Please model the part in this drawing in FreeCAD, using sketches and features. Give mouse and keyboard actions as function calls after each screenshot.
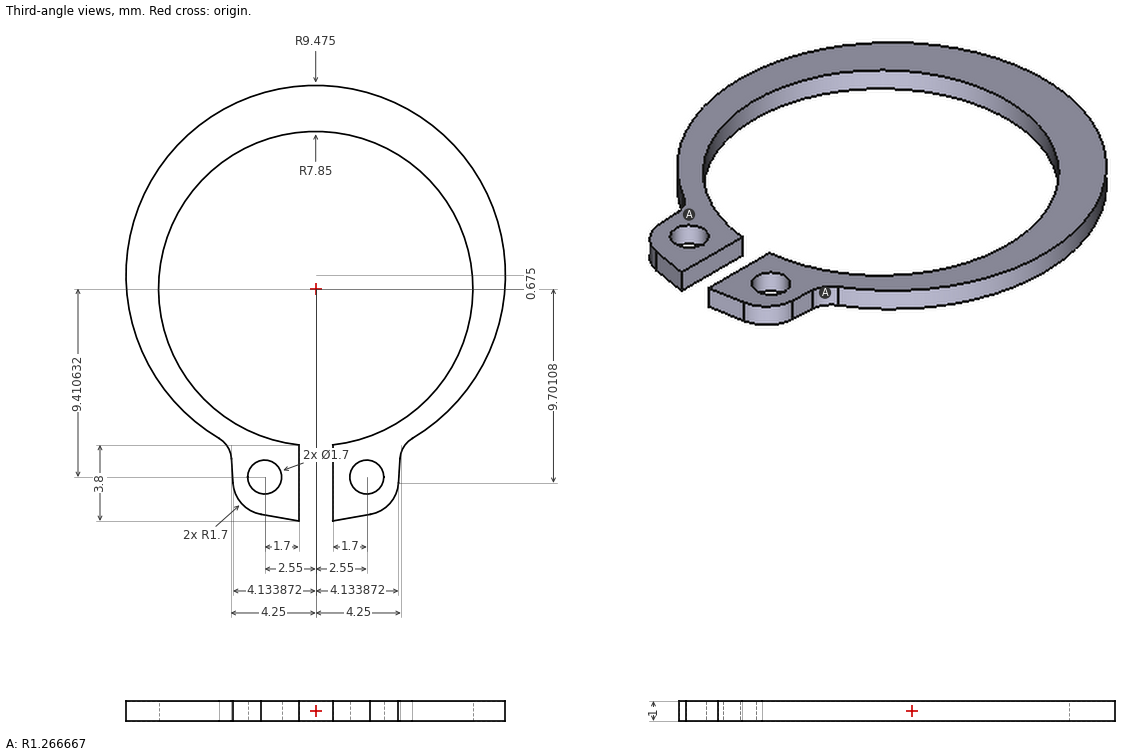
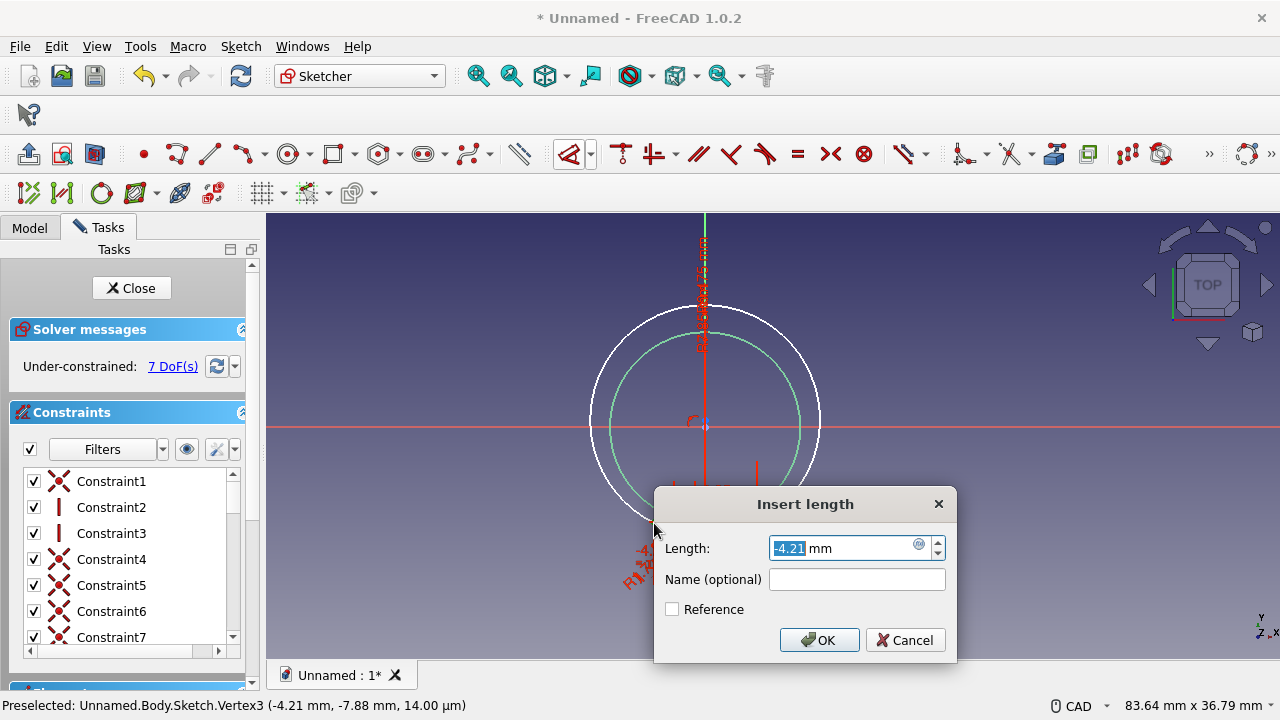
text(-4.25)
key(Return)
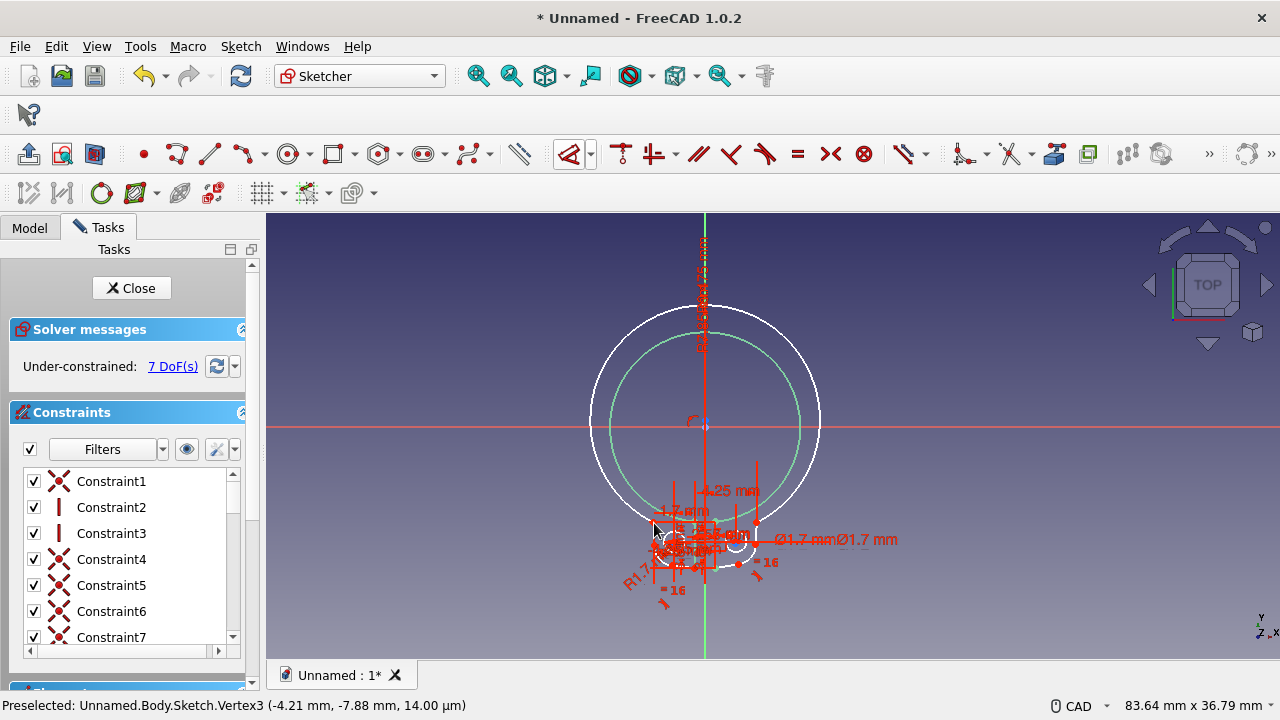
scroll(705, 420, up, 8)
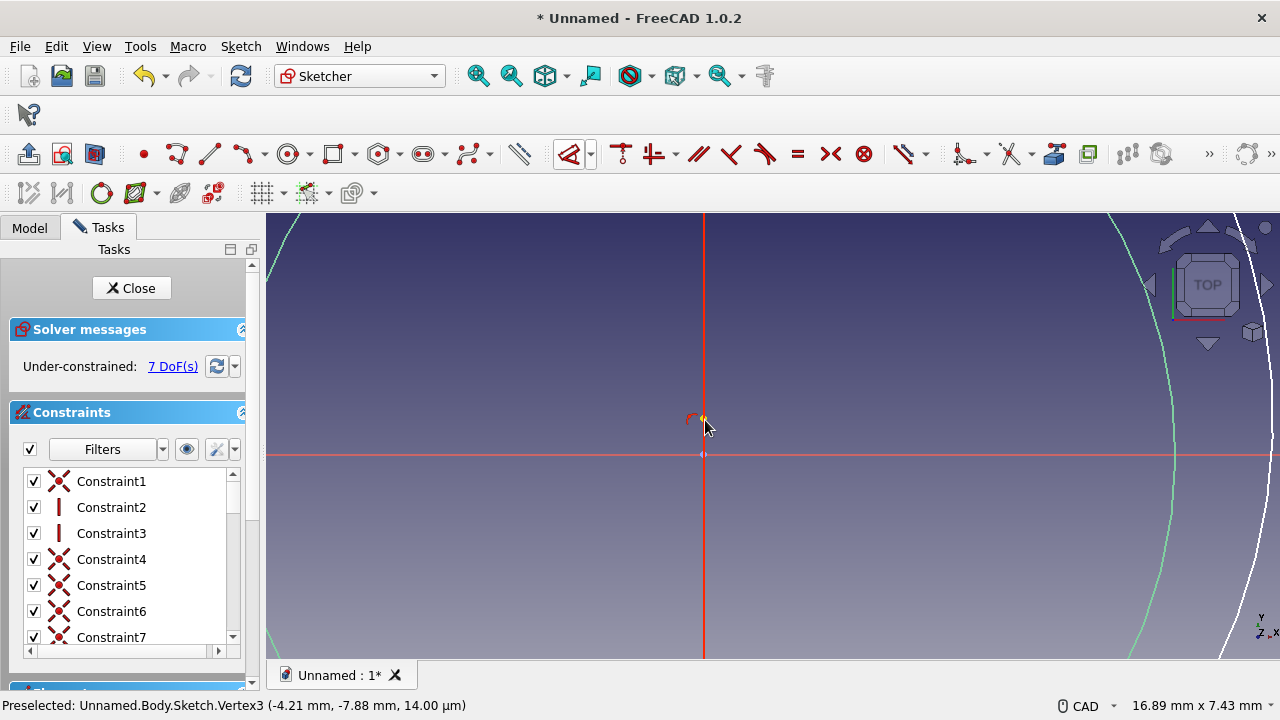
click(704, 418)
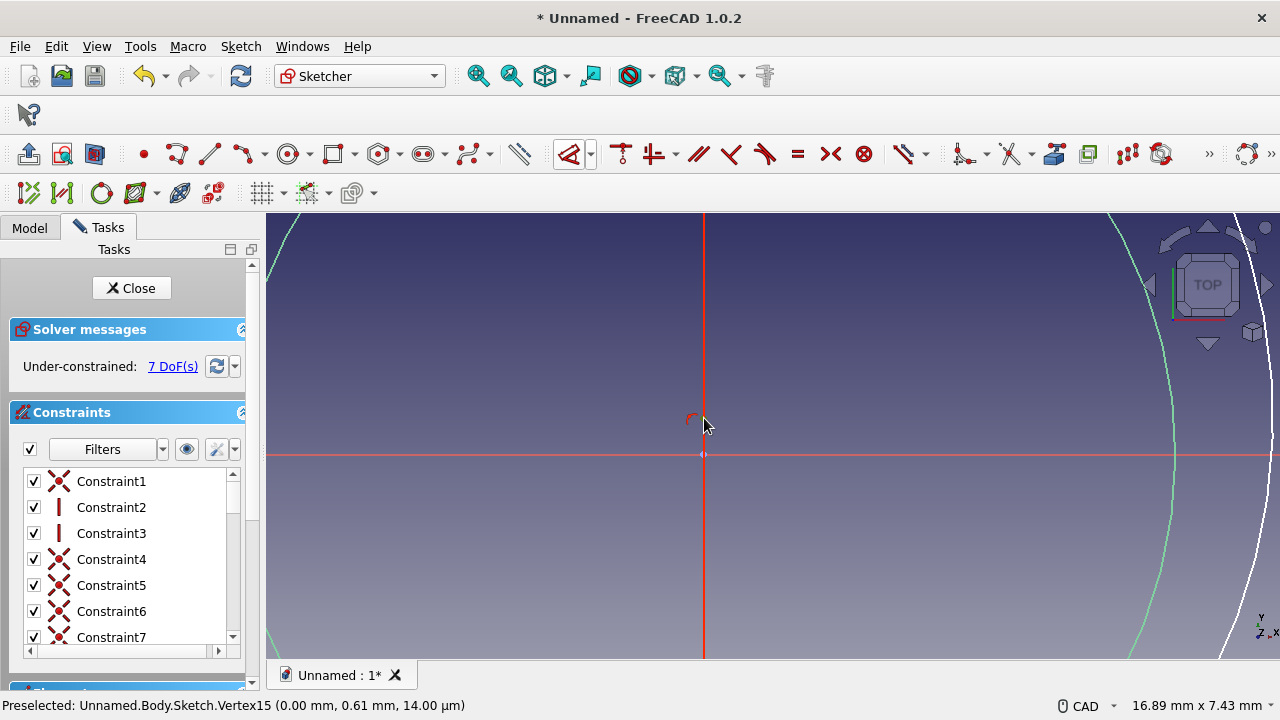
key(i)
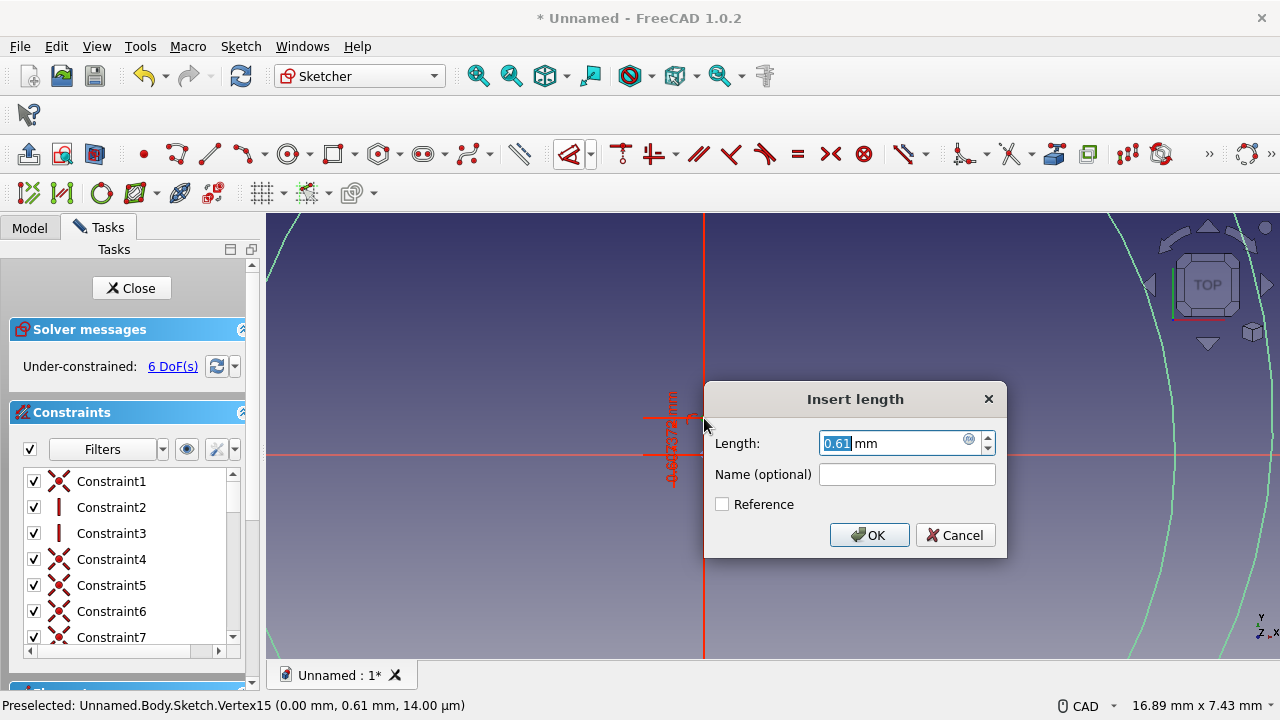
text(0.675)
key(Return)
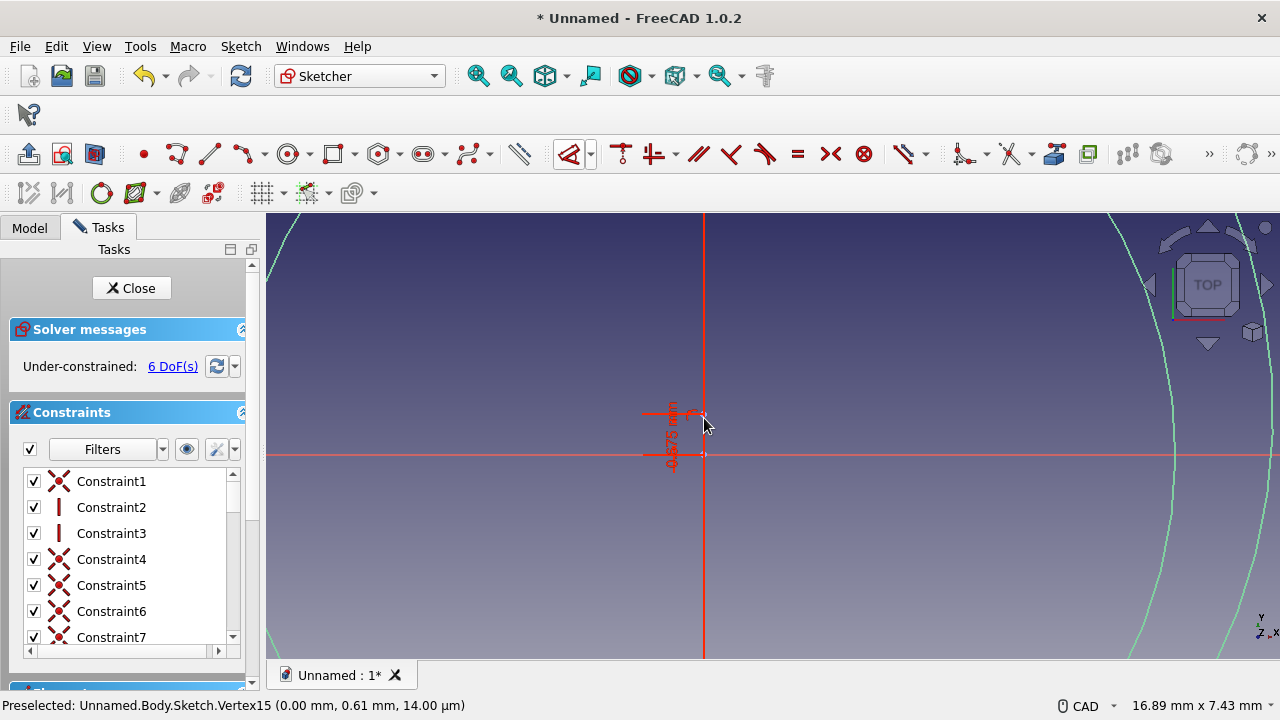
scroll(705, 420, down, 8)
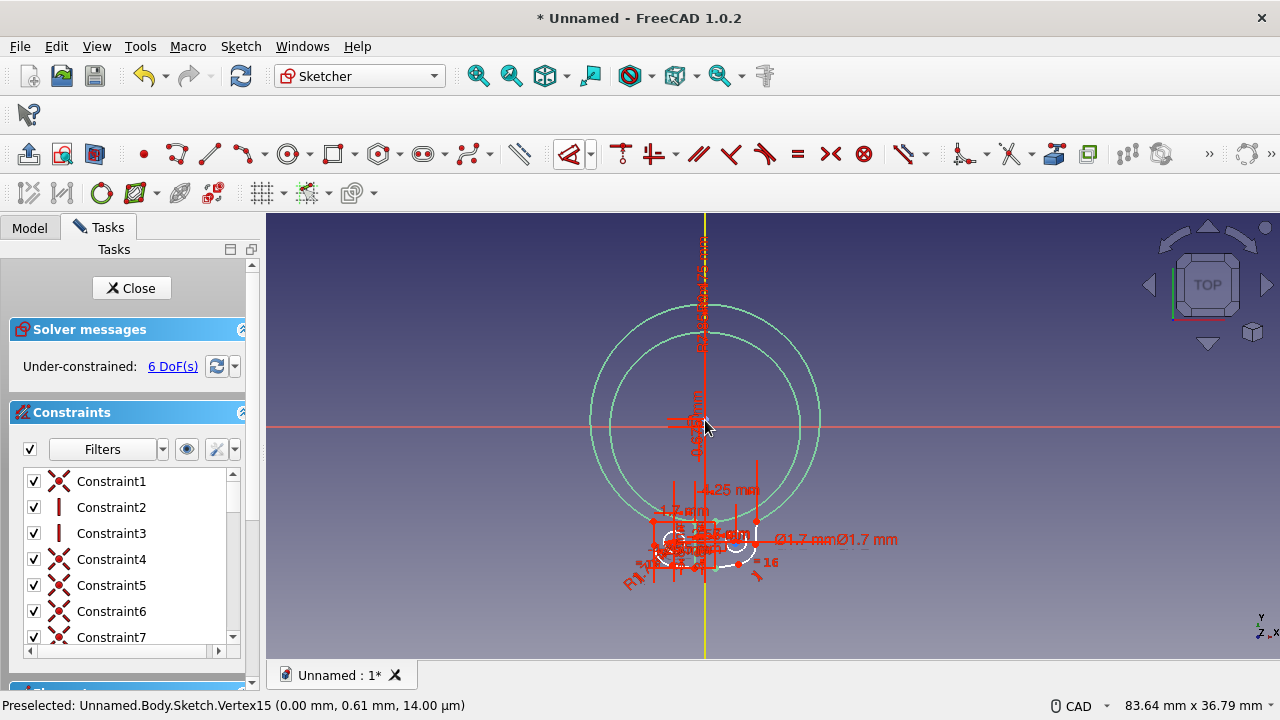
click(756, 545)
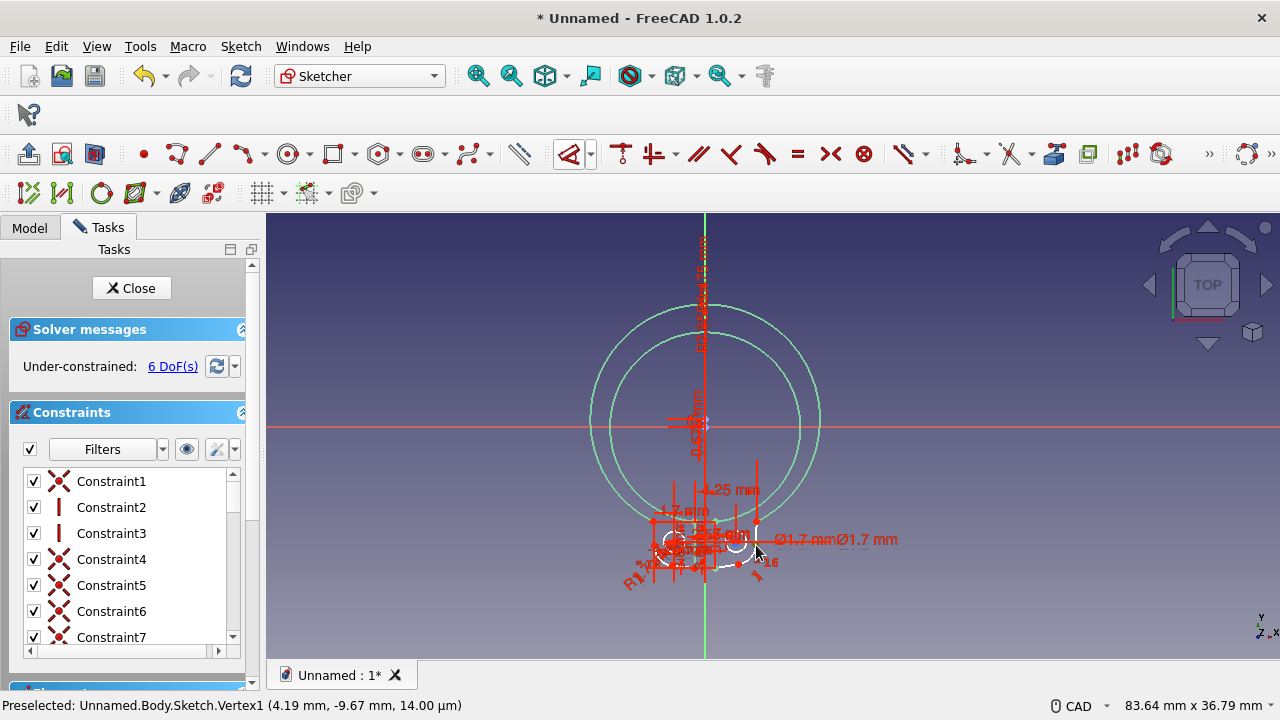
click(590, 154)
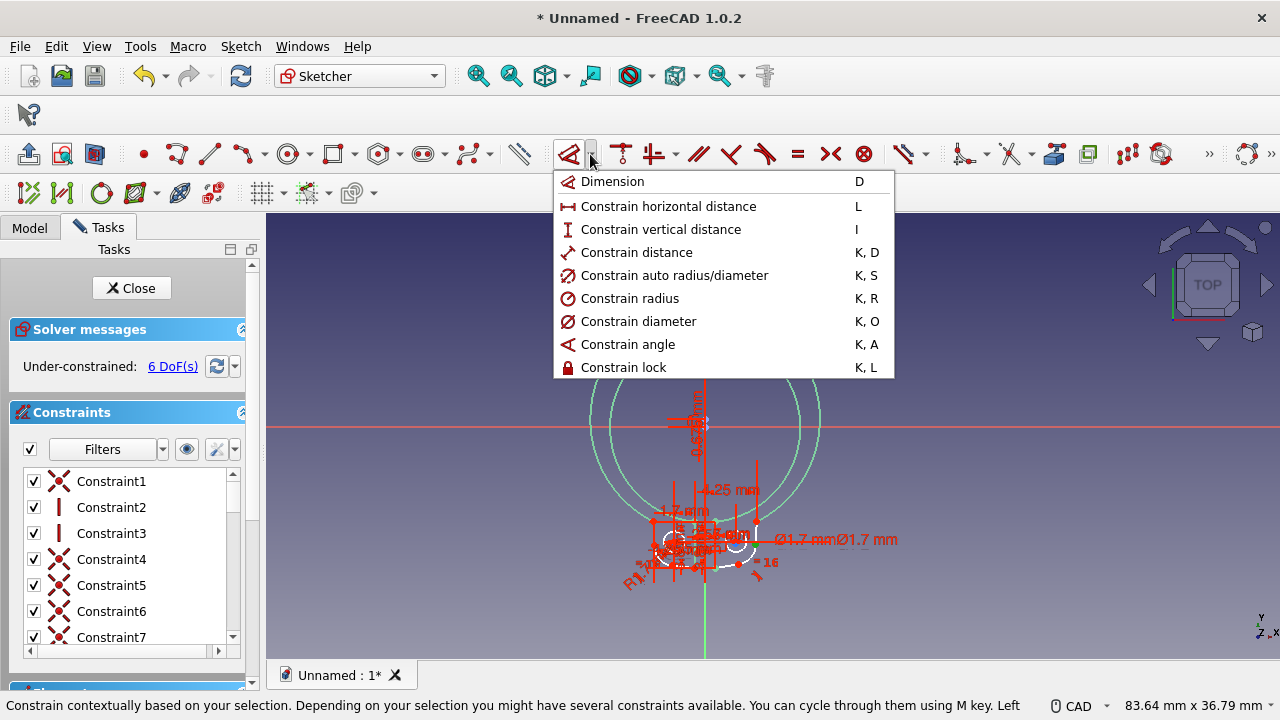
click(724, 230)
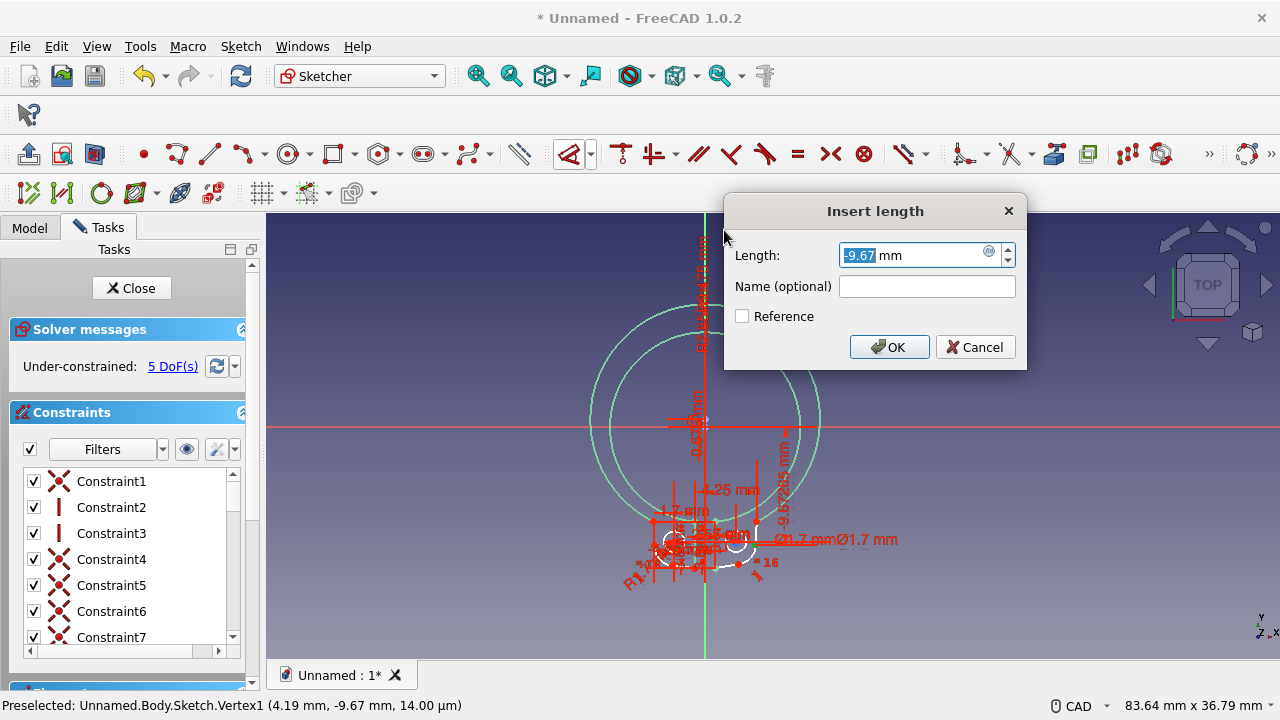
text(-9.70108)
key(Return)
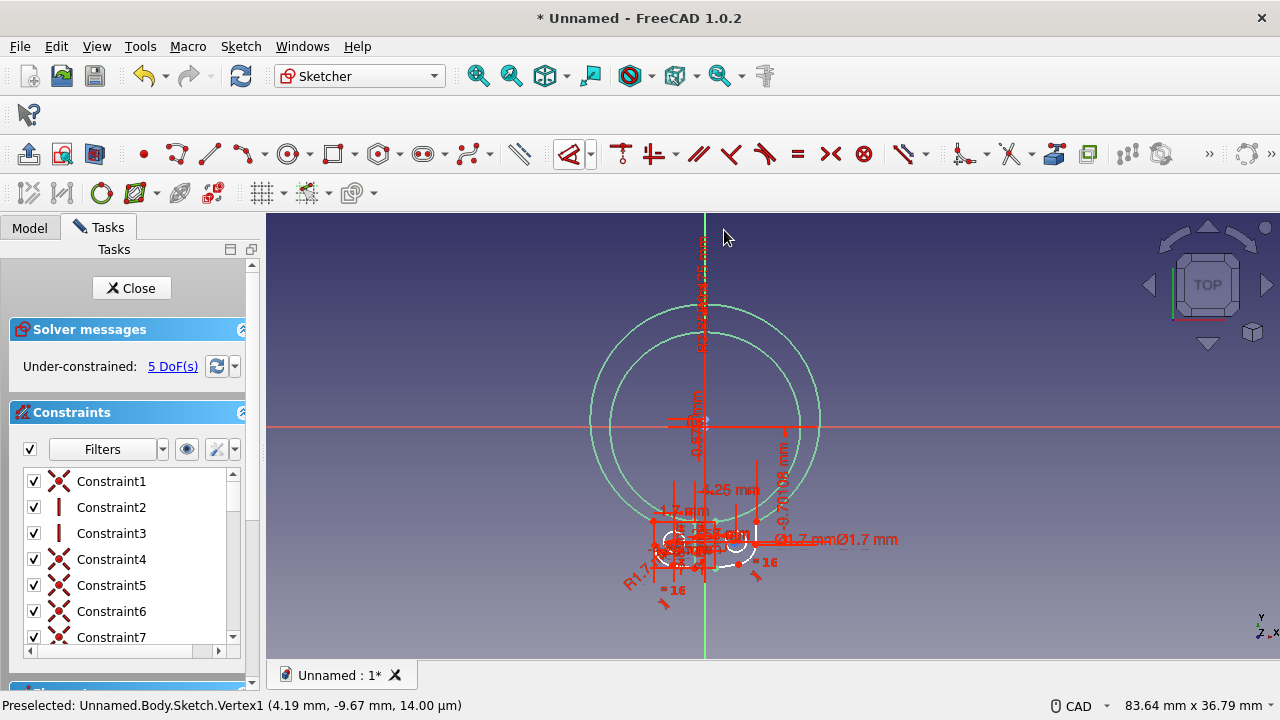
click(654, 546)